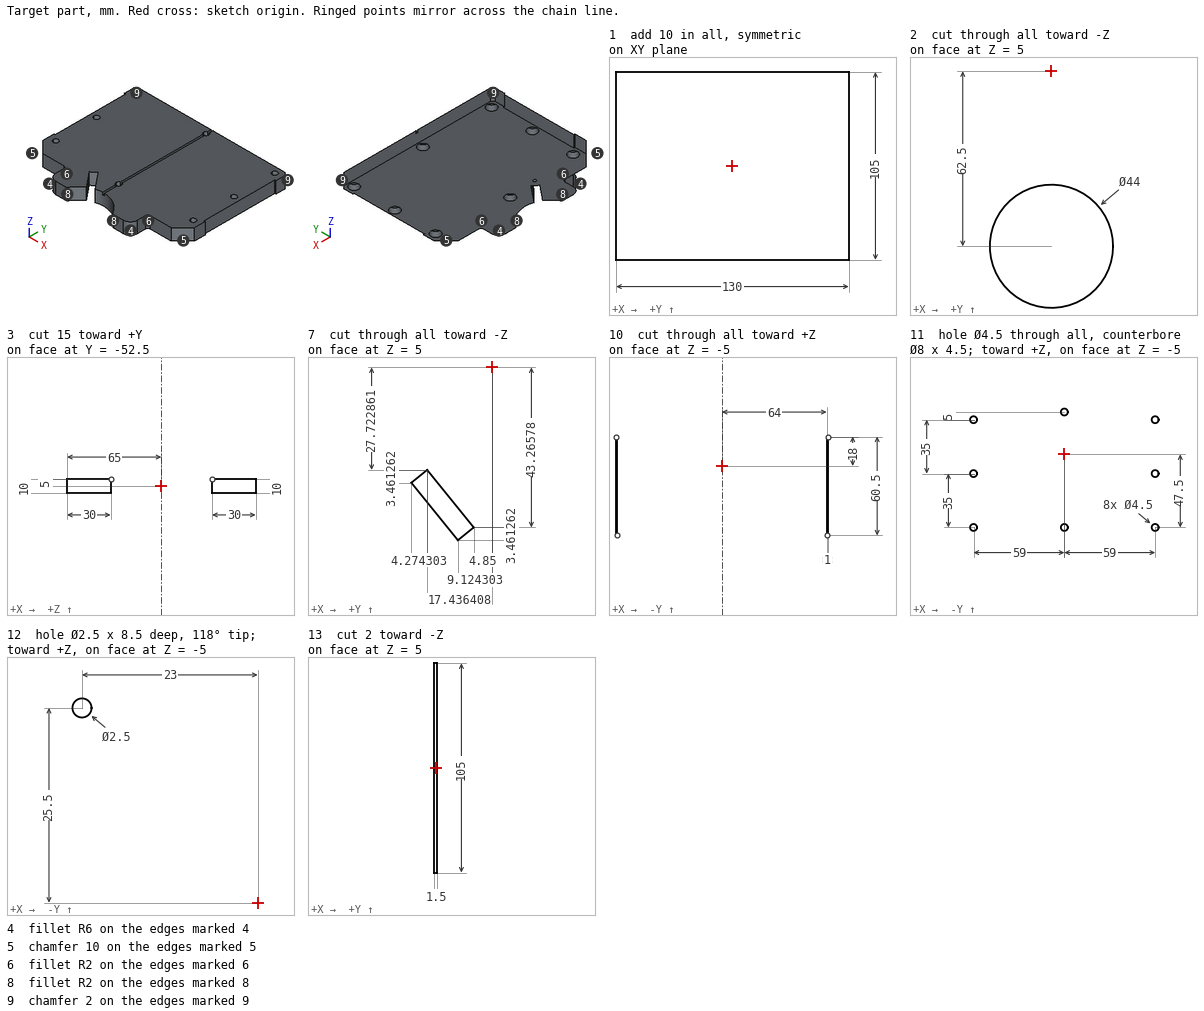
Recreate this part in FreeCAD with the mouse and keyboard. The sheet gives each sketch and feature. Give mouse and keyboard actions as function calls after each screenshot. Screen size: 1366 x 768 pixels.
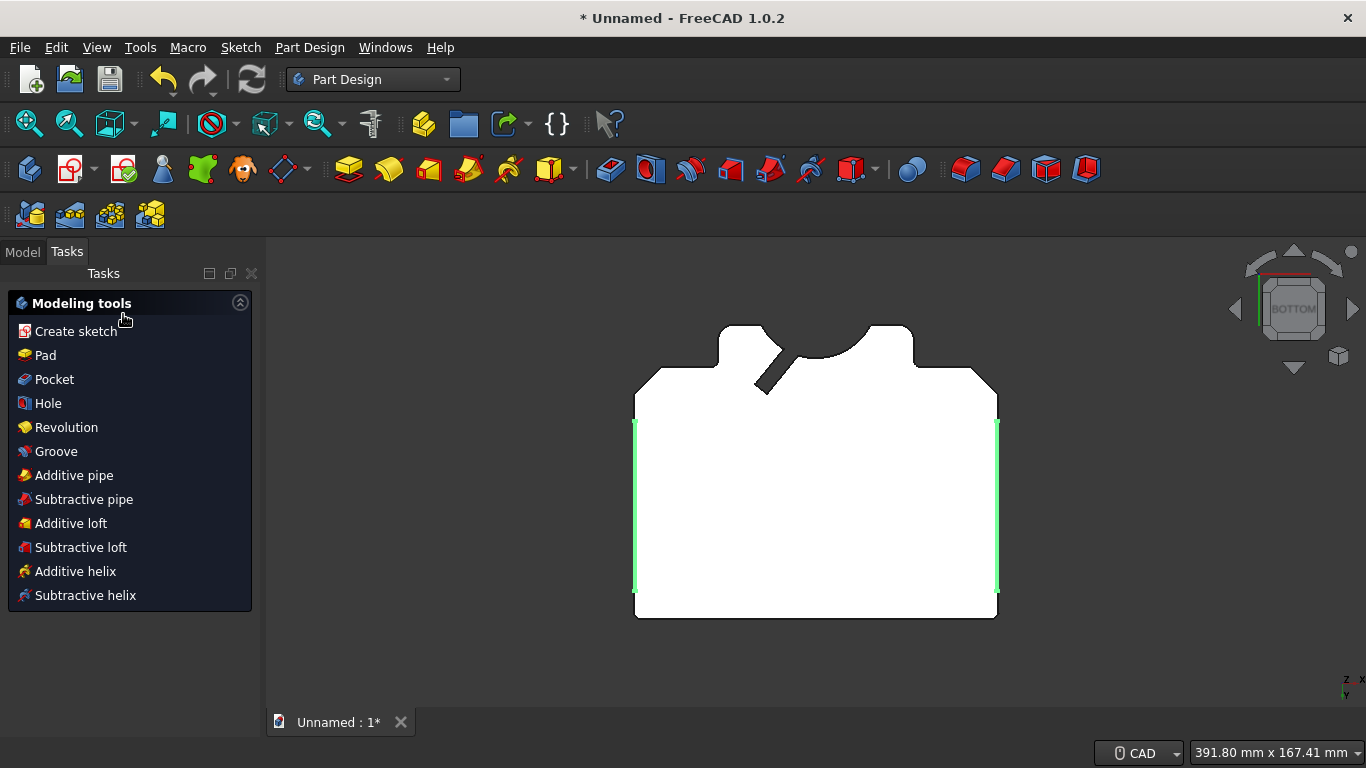
click(612, 170)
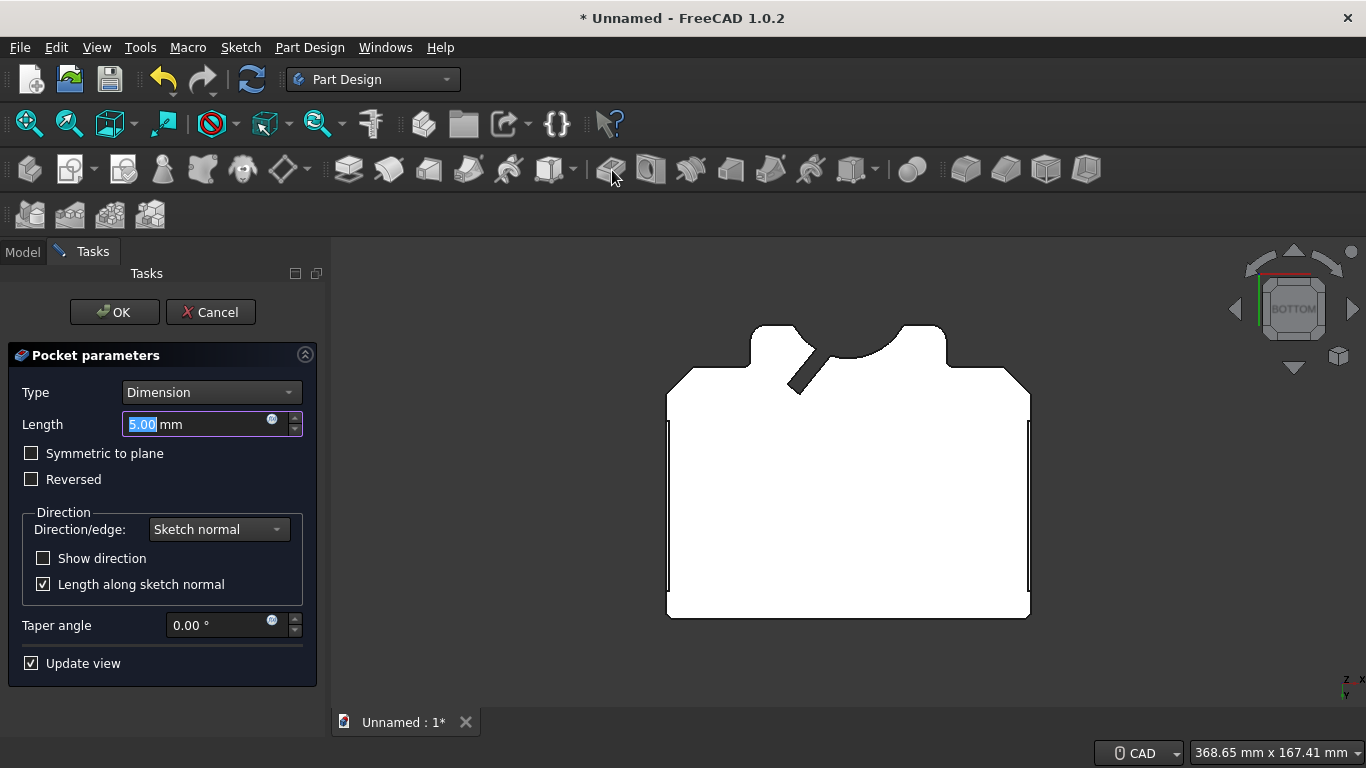
click(212, 392)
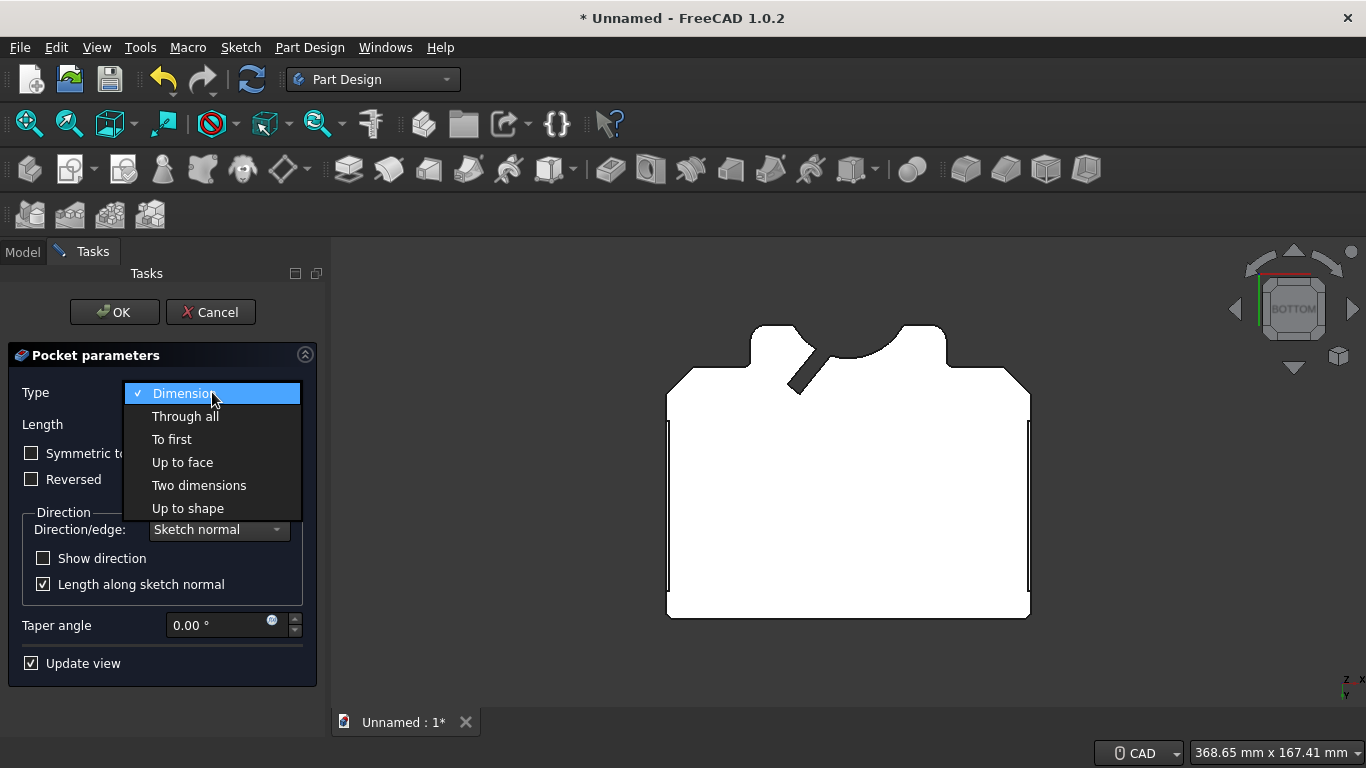
click(212, 416)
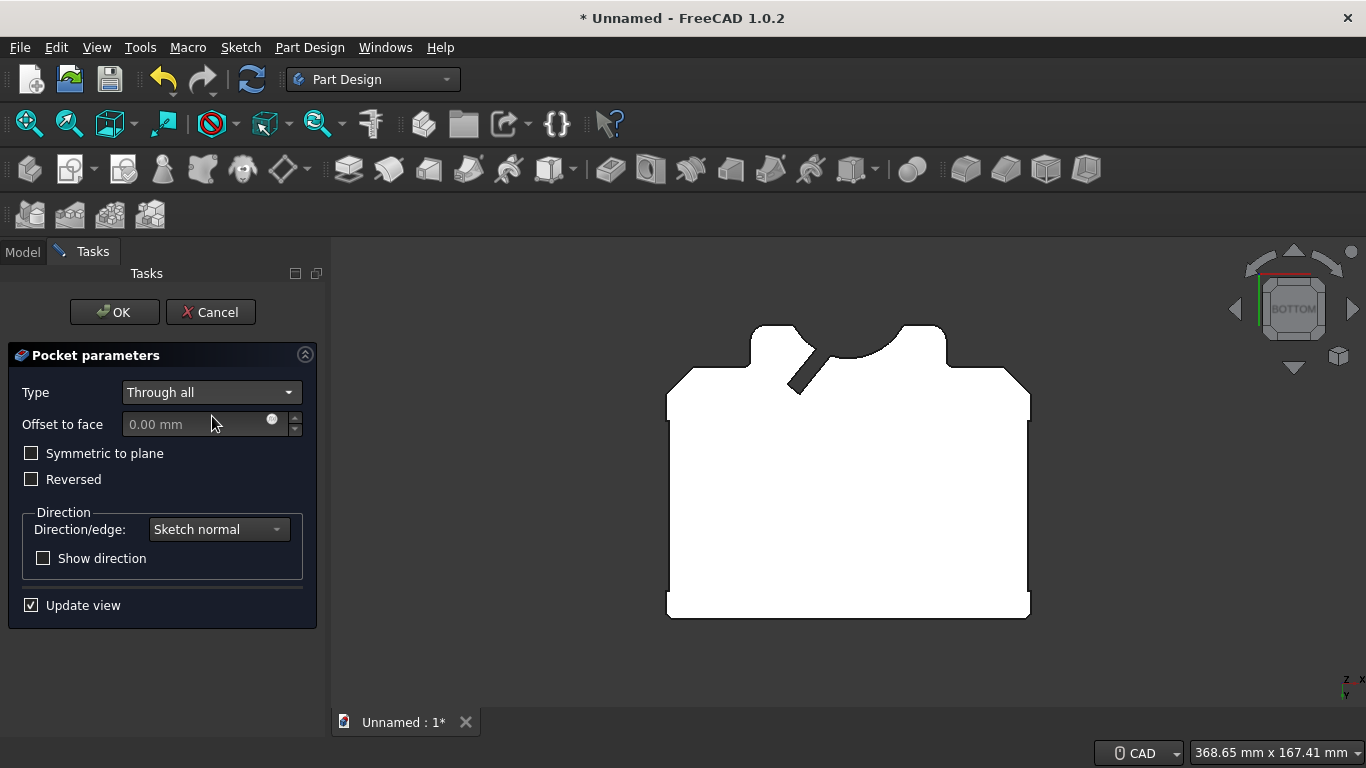
click(115, 312)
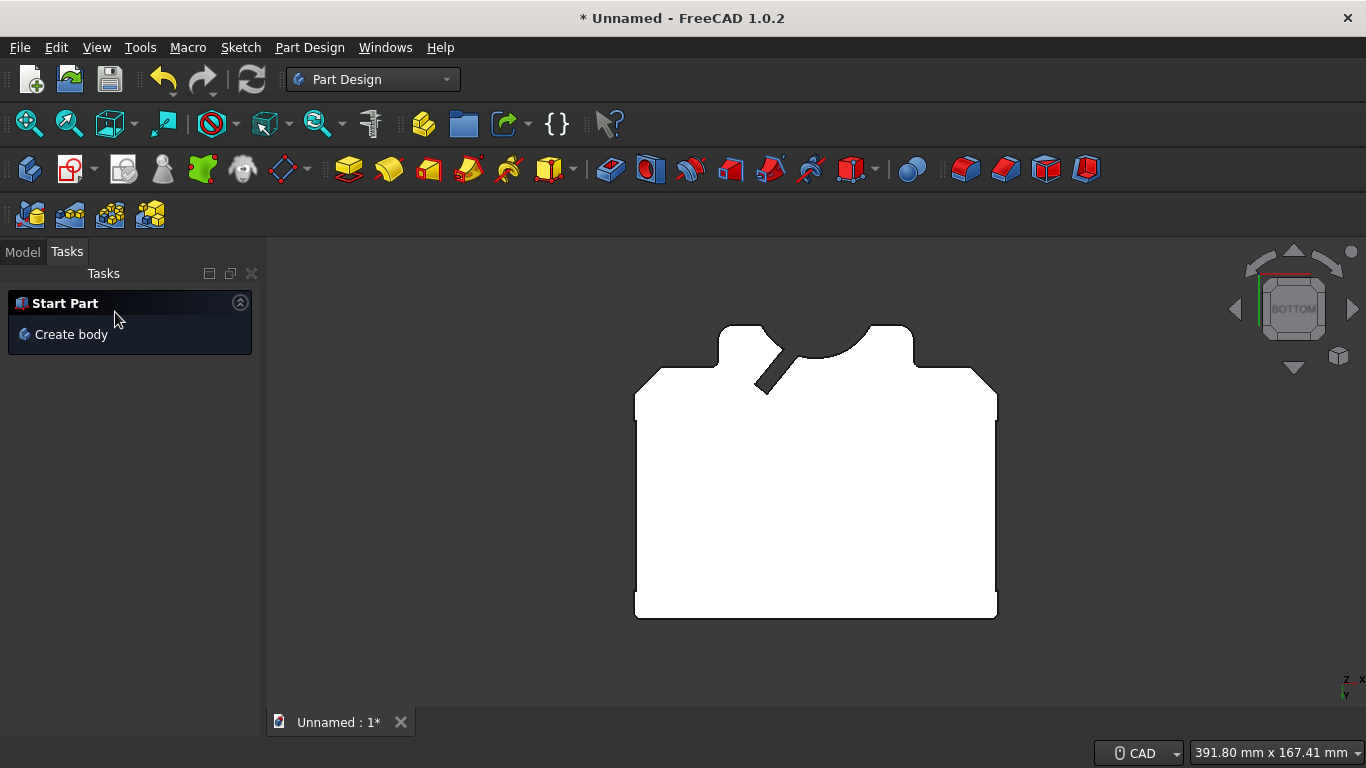
click(868, 471)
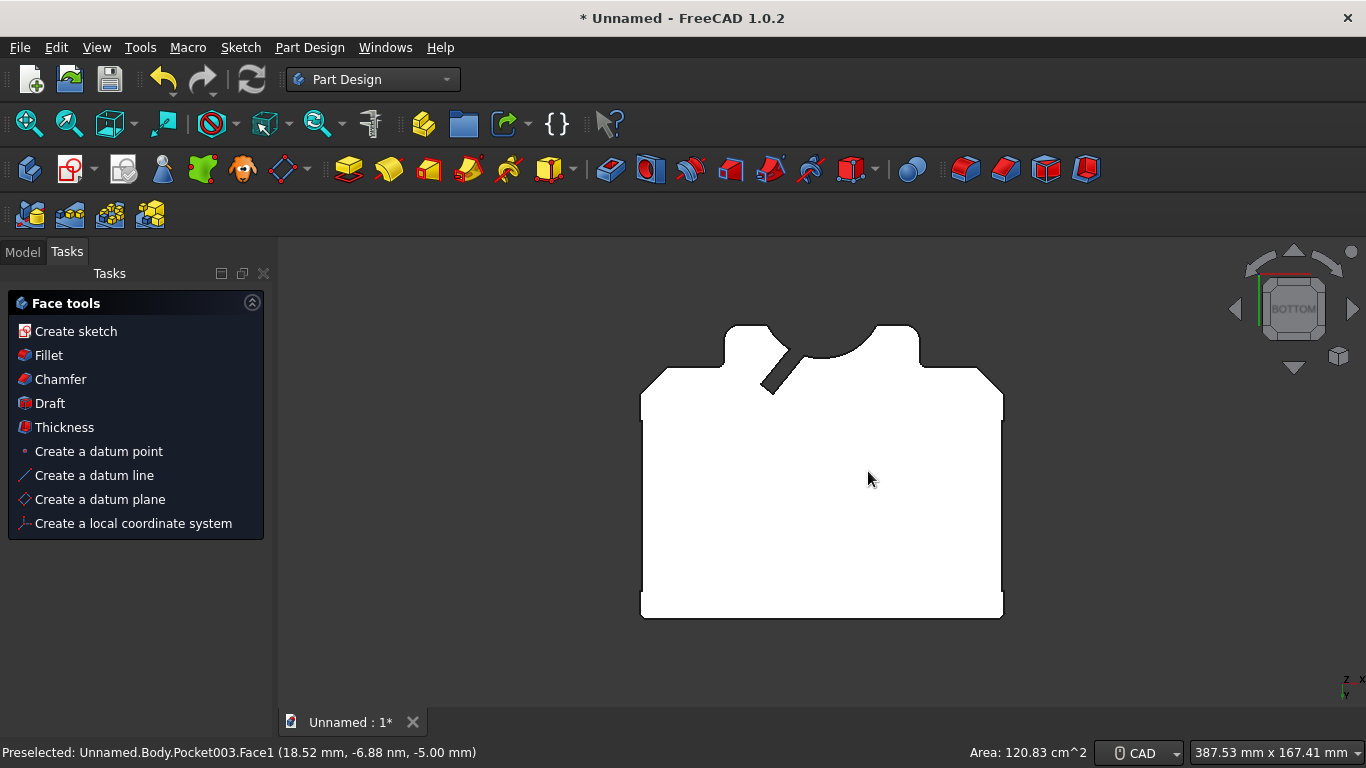
click(70, 170)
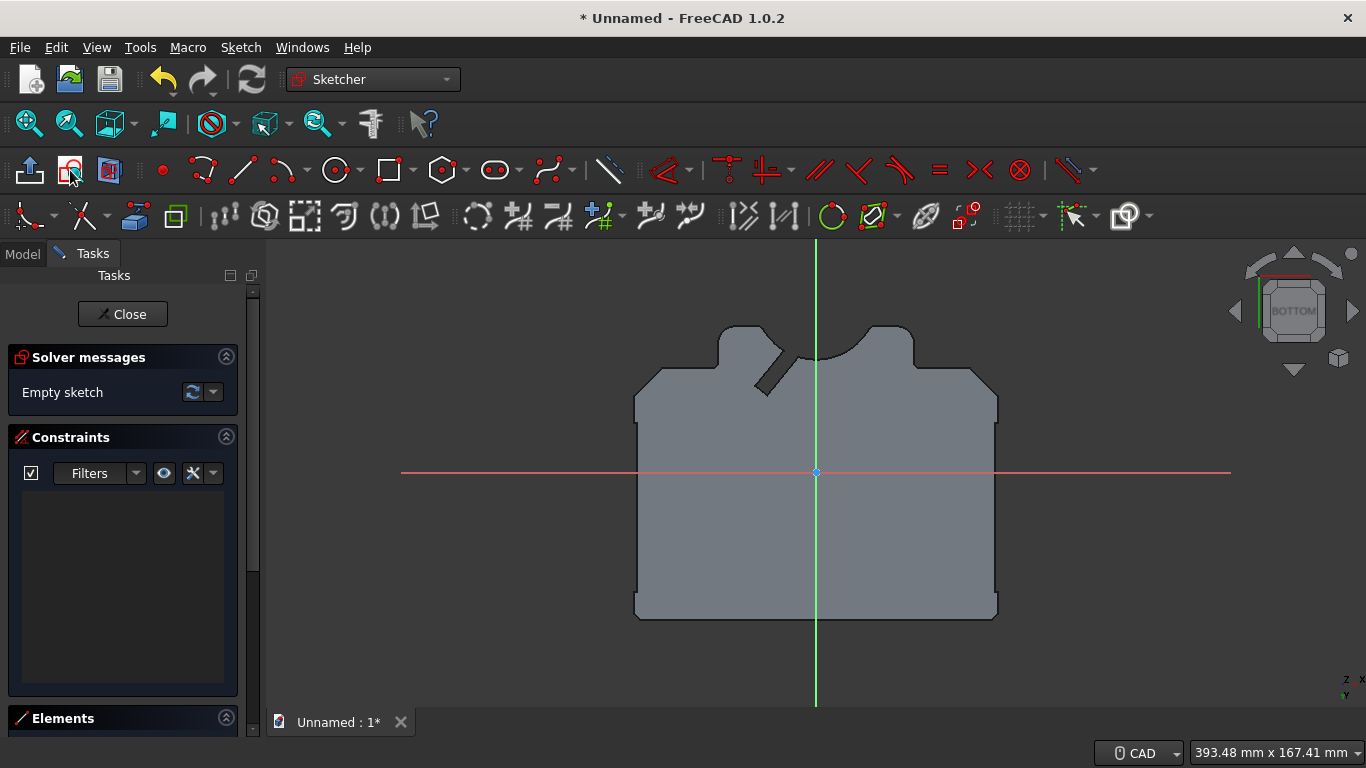
click(336, 170)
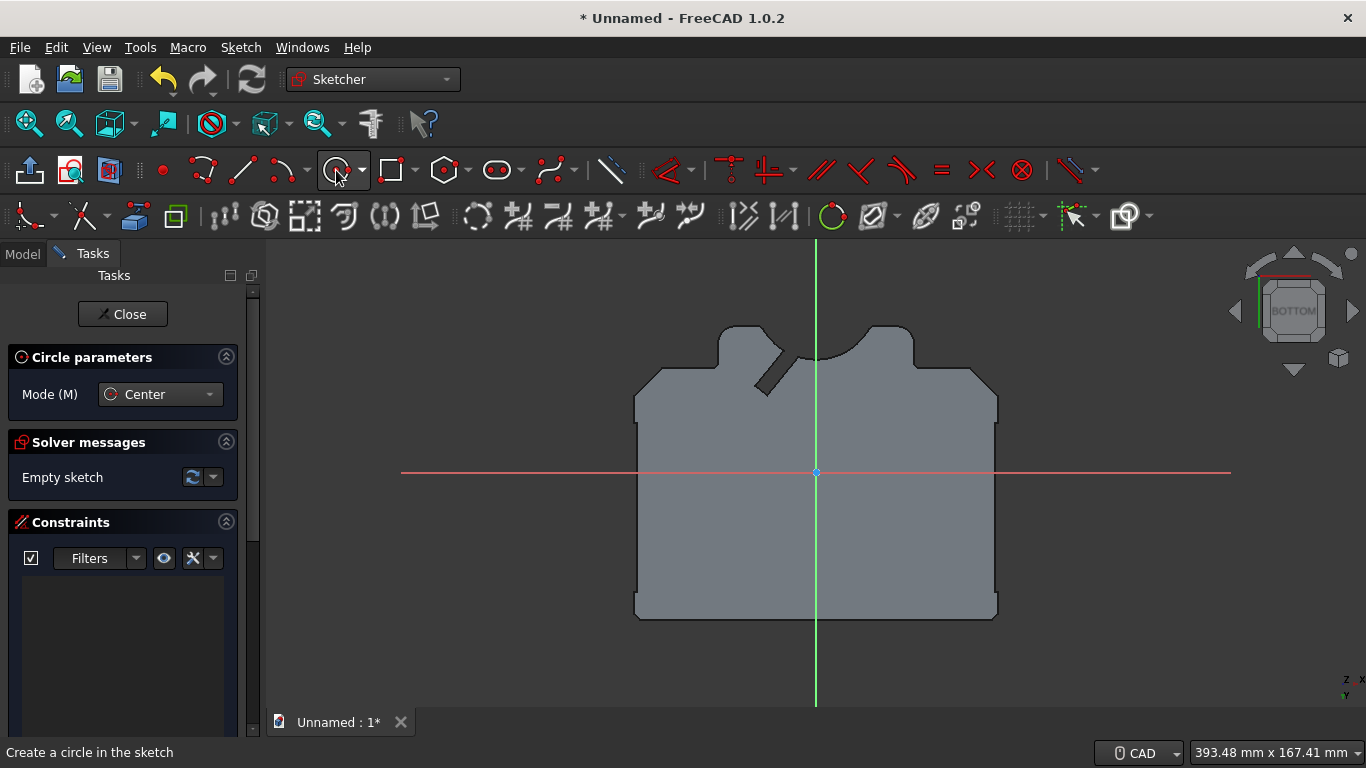
scroll(981, 606, up, 7)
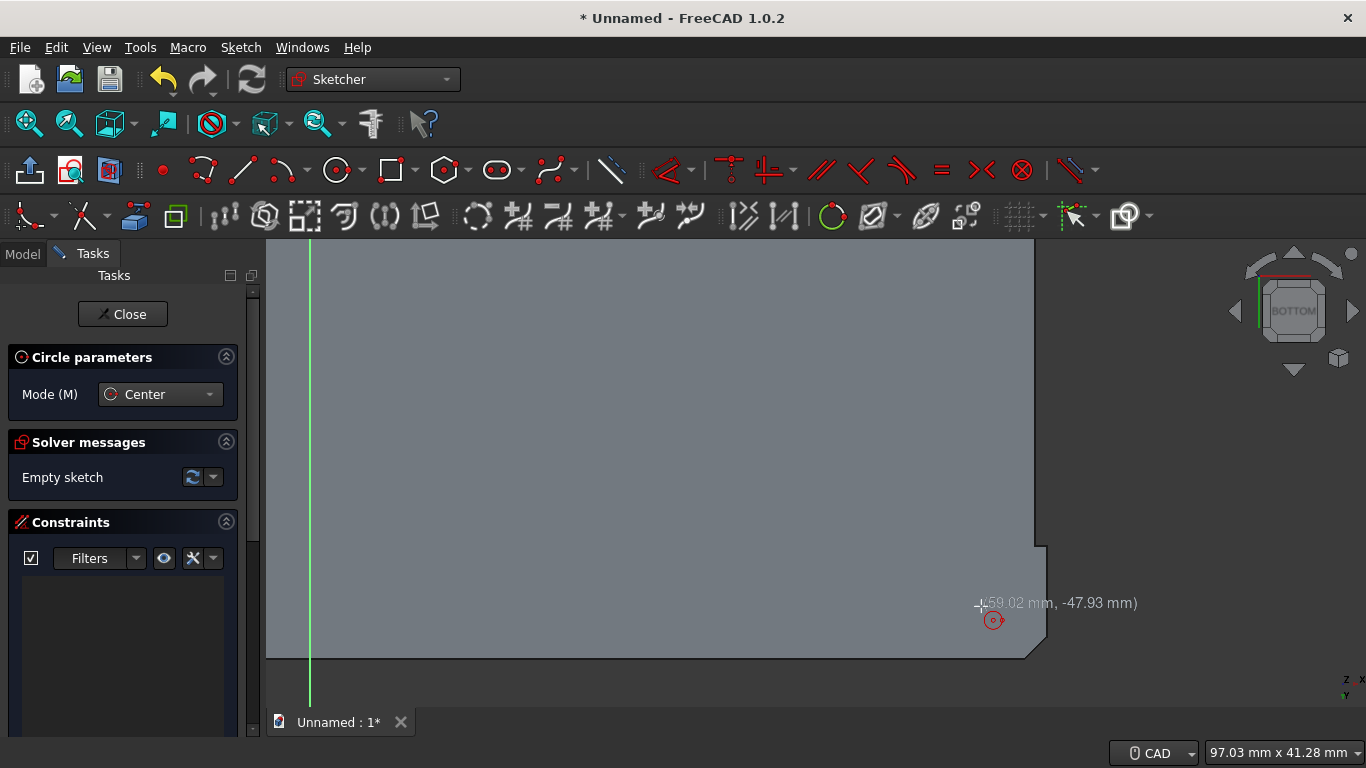
scroll(936, 600, down, 6)